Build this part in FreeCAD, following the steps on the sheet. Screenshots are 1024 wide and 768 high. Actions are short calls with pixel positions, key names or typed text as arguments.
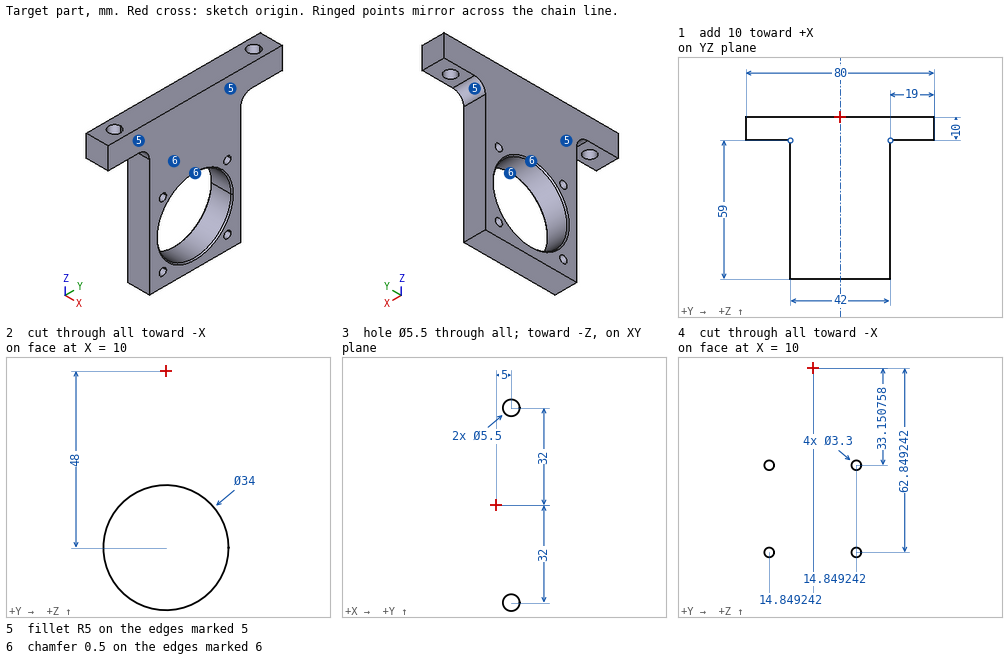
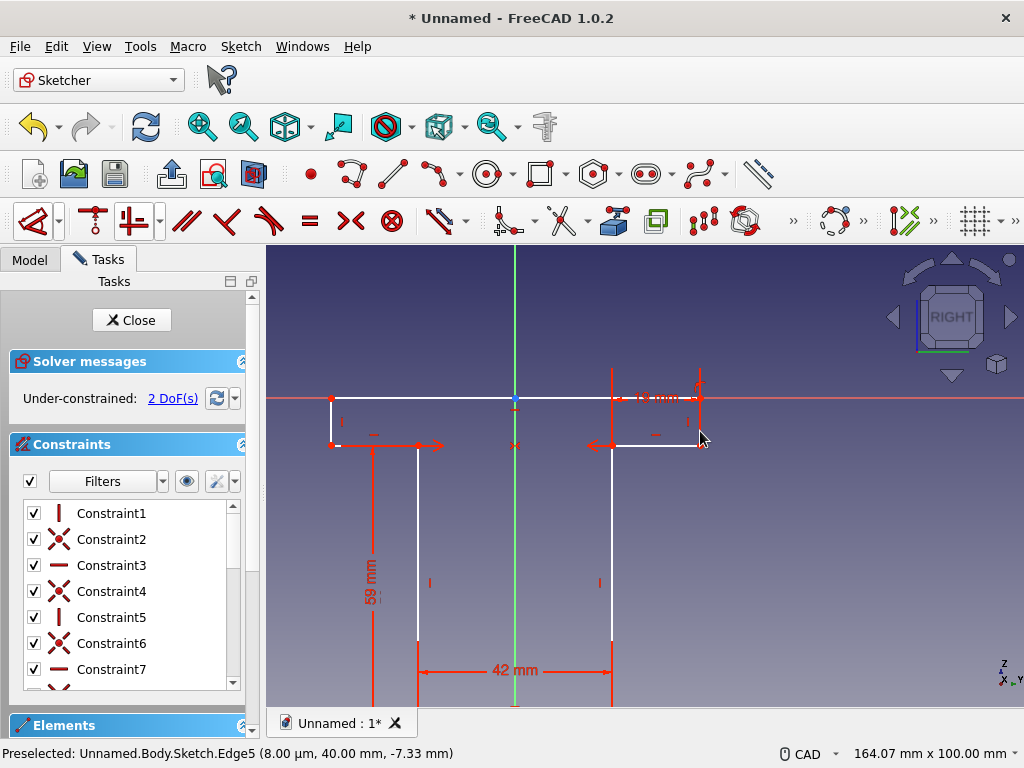
click(58, 222)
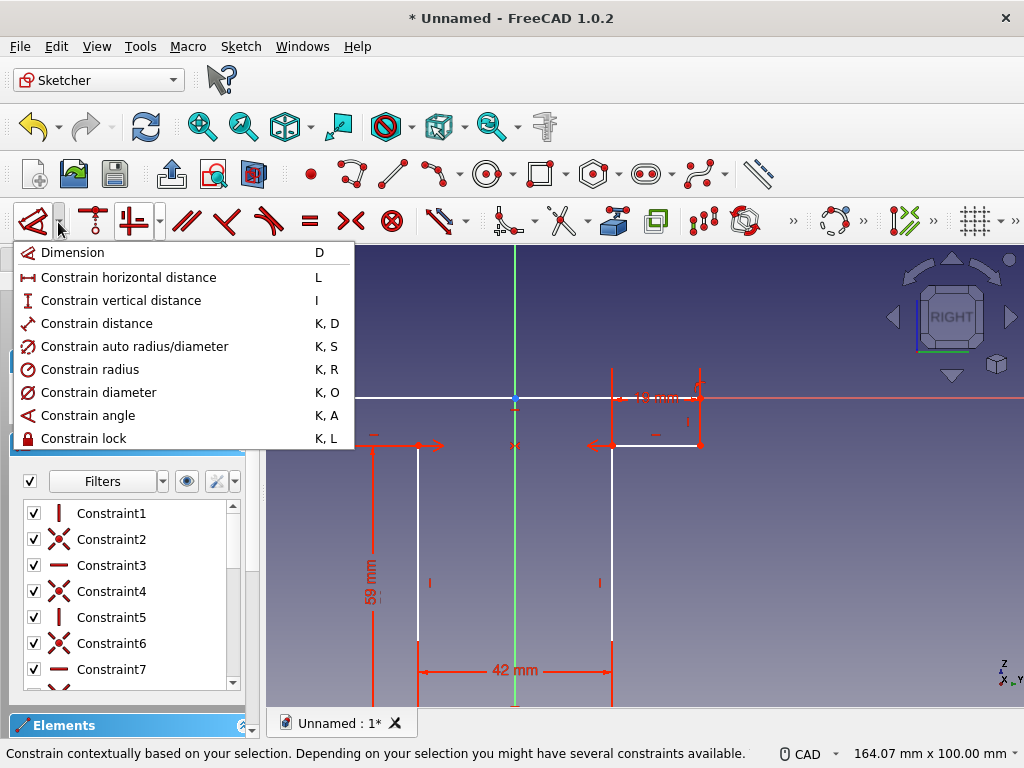
click(184, 300)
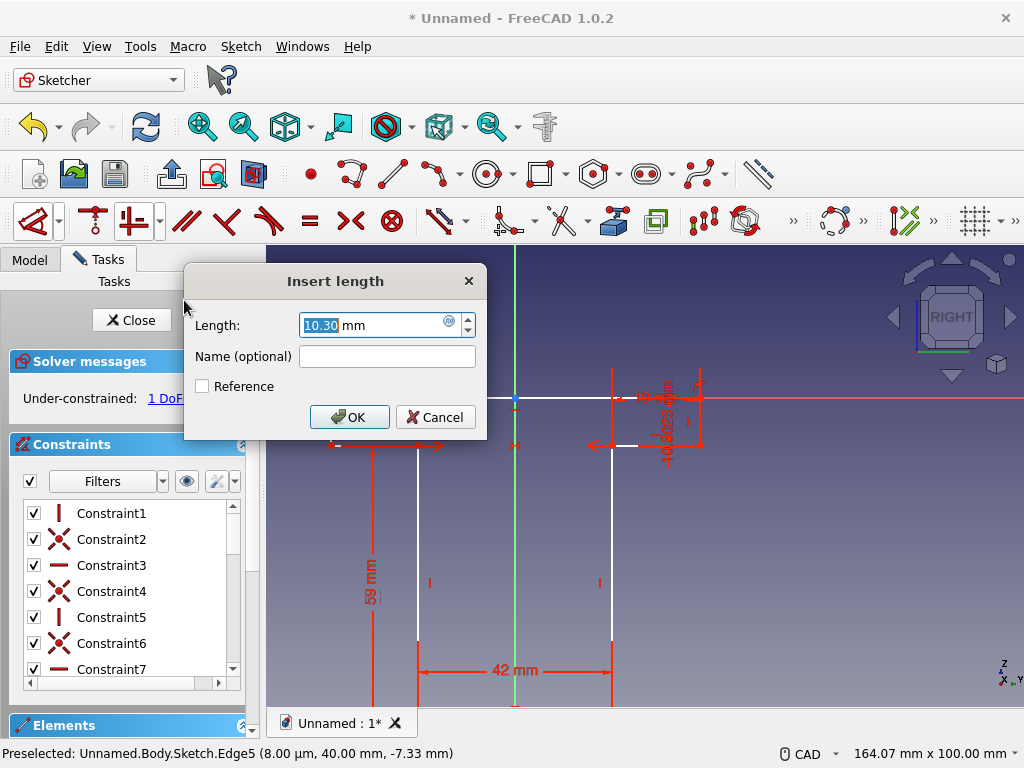
text(10)
key(Return)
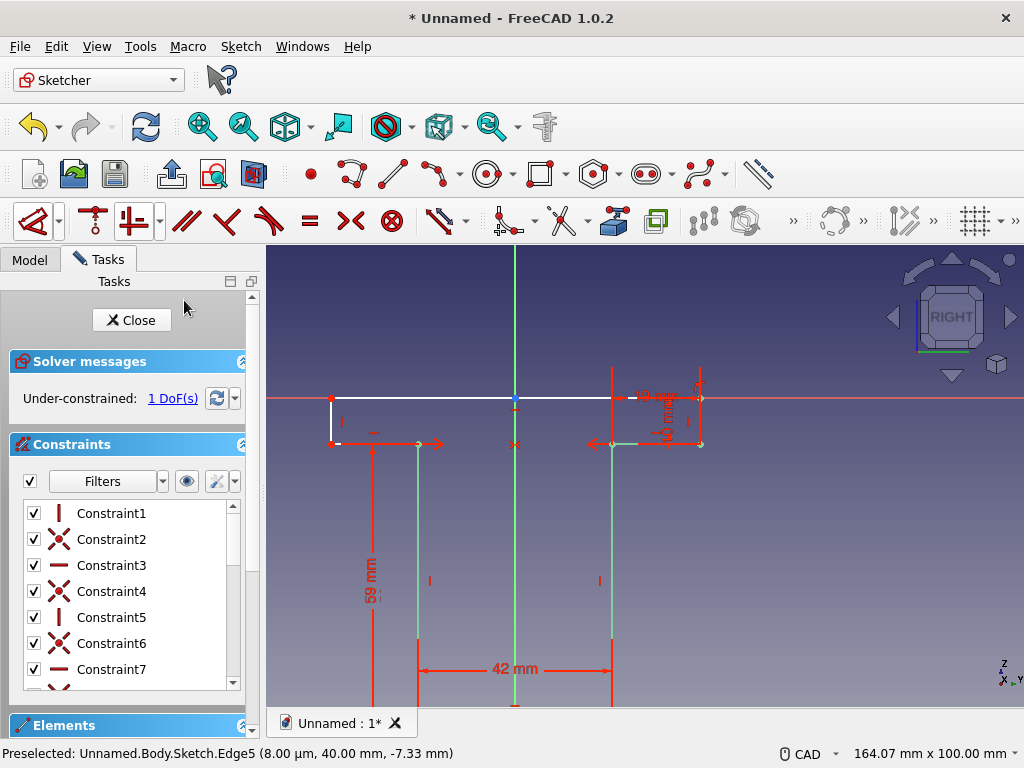
click(590, 398)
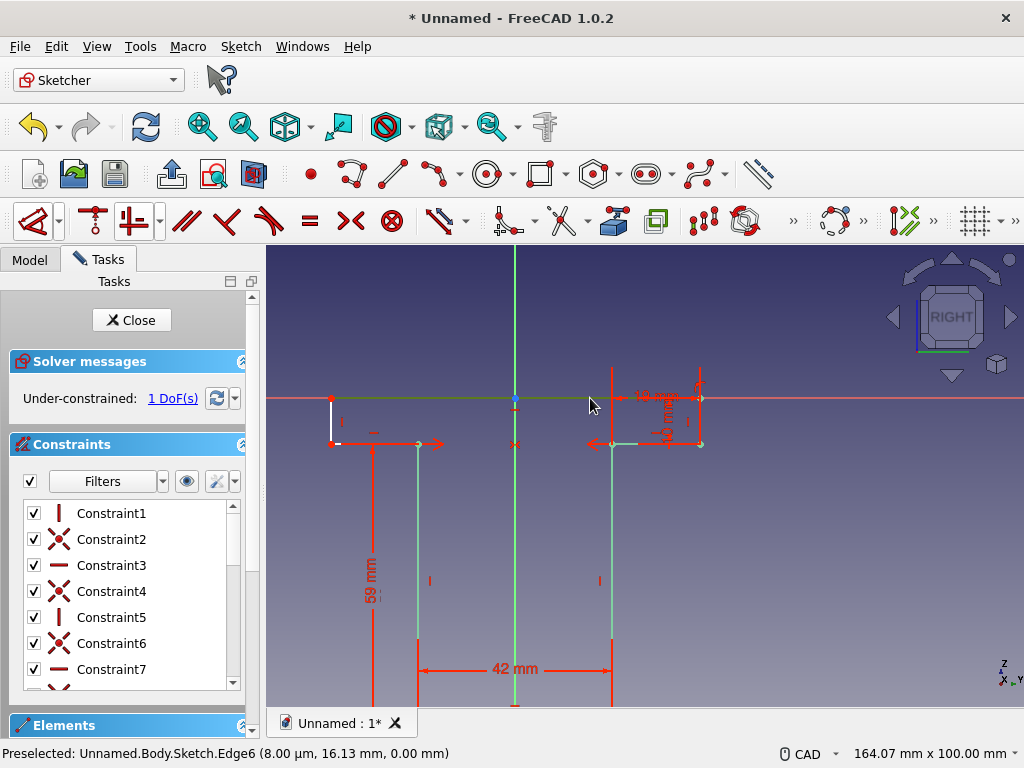
key(l)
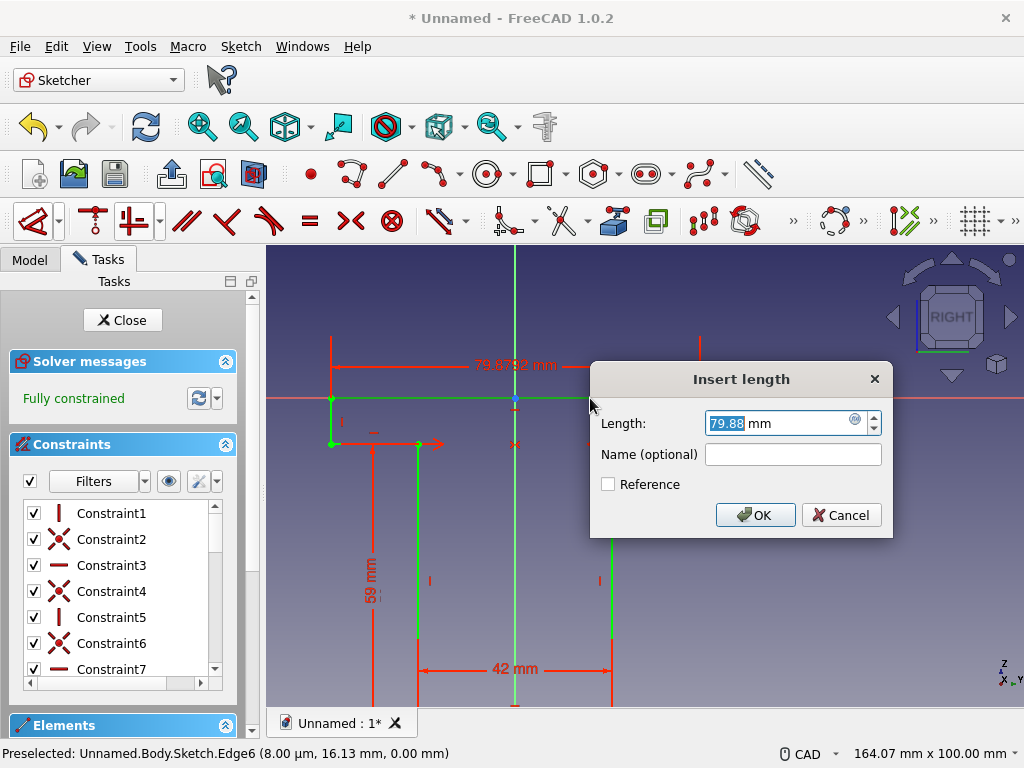
text(80)
key(Return)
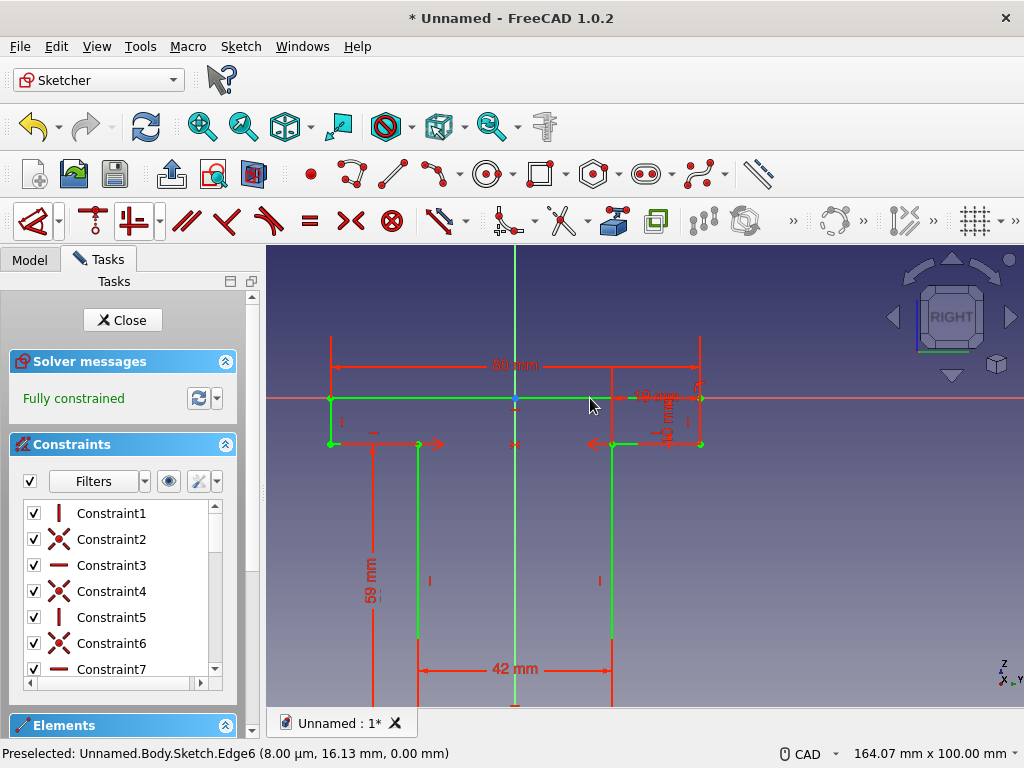
click(123, 320)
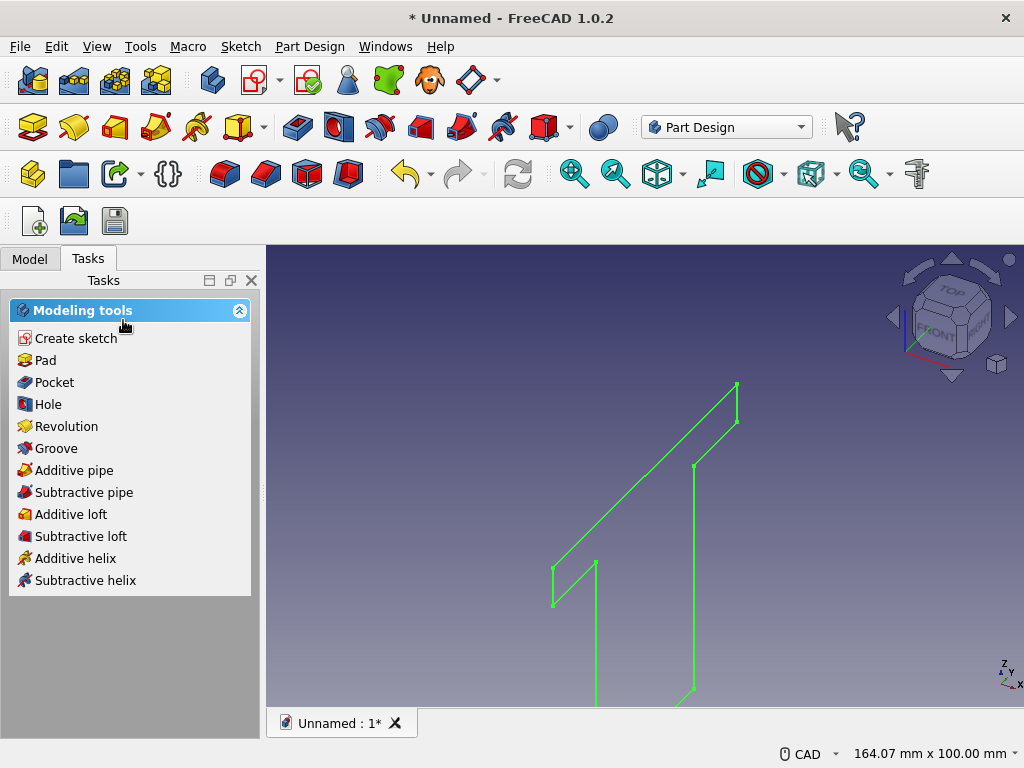
click(33, 128)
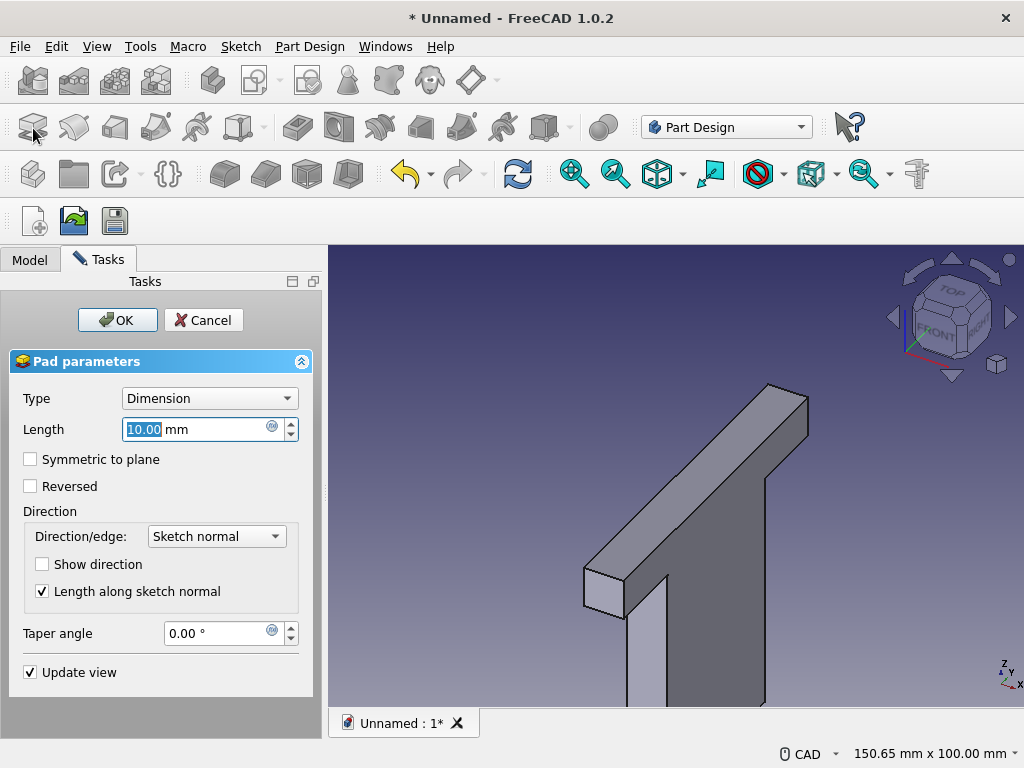
text(10)
key(Tab)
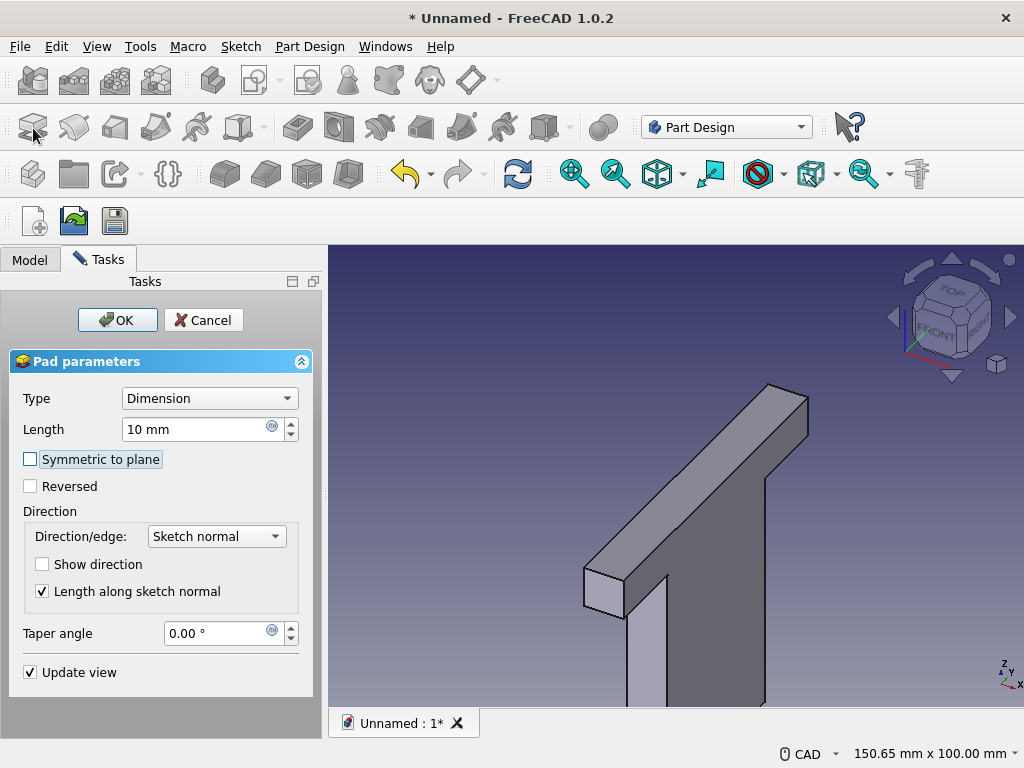
click(118, 320)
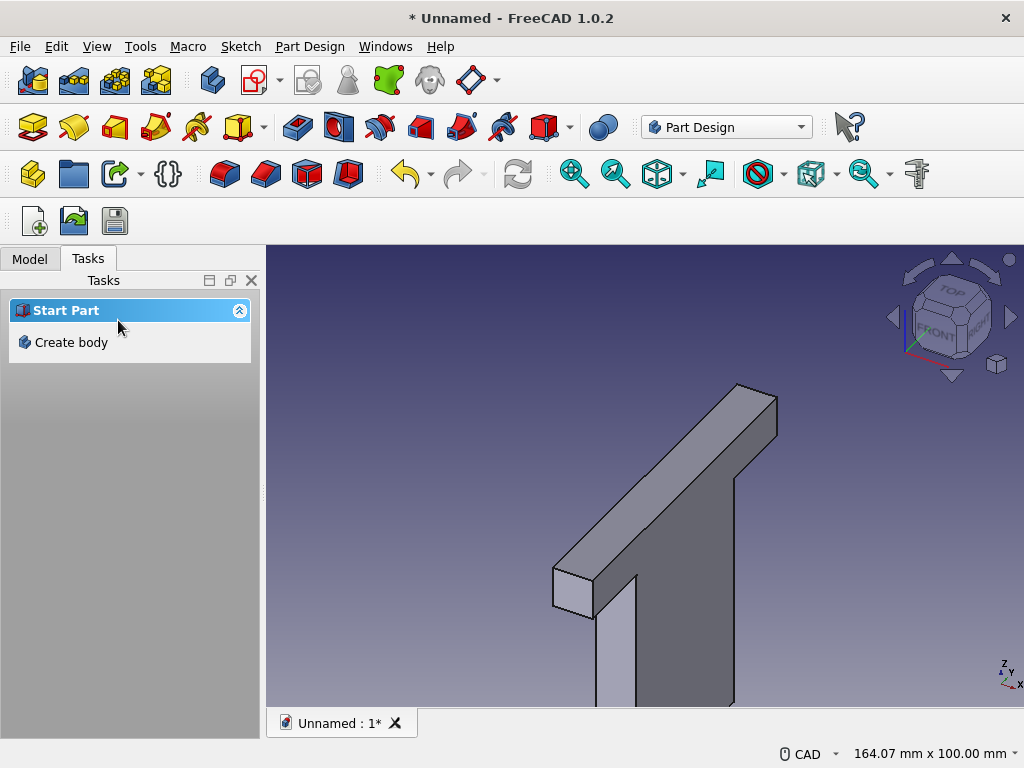
click(575, 174)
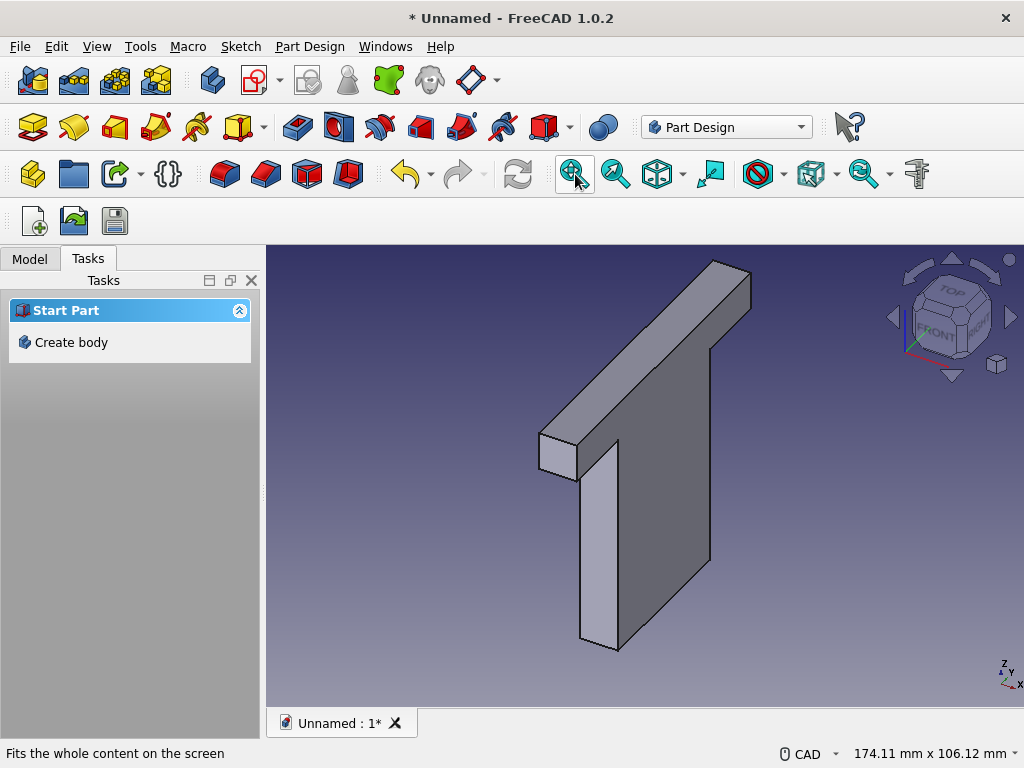
click(664, 516)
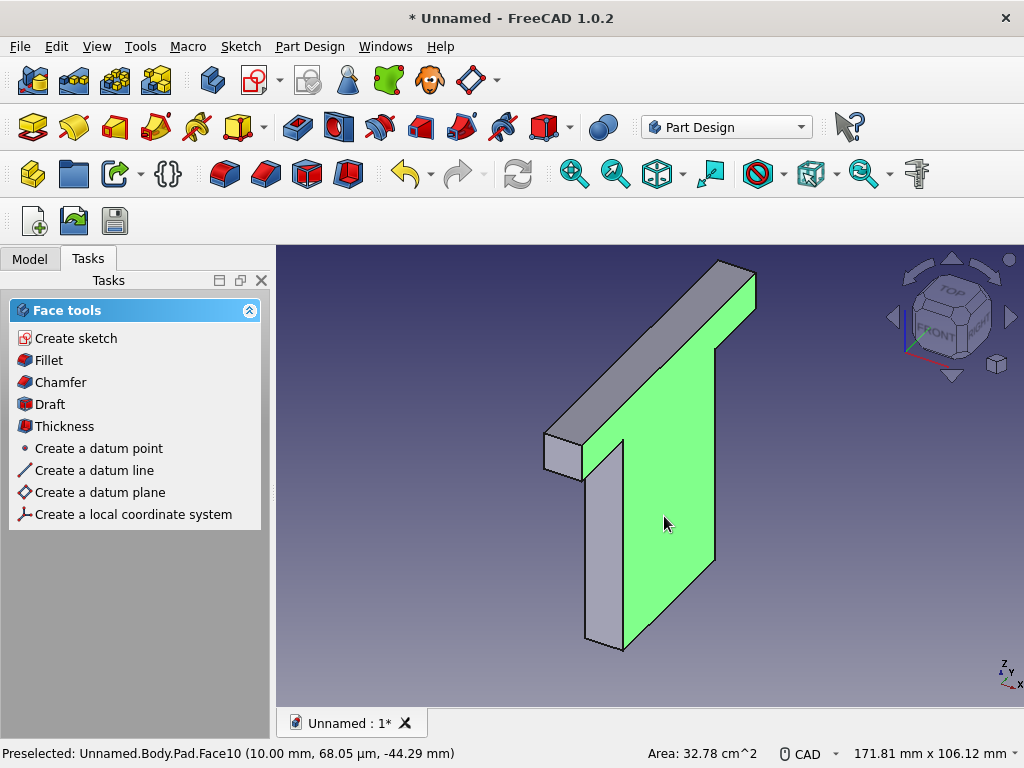
click(254, 80)